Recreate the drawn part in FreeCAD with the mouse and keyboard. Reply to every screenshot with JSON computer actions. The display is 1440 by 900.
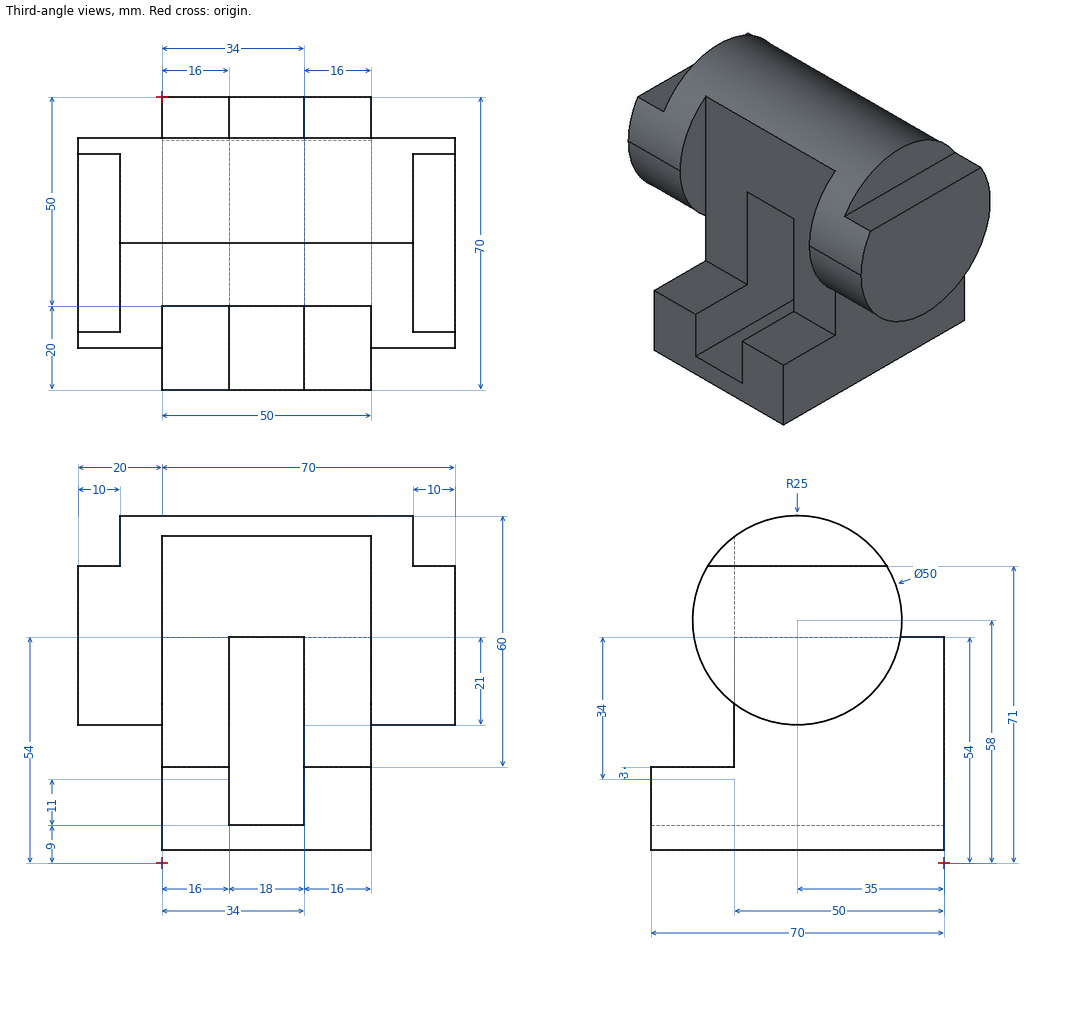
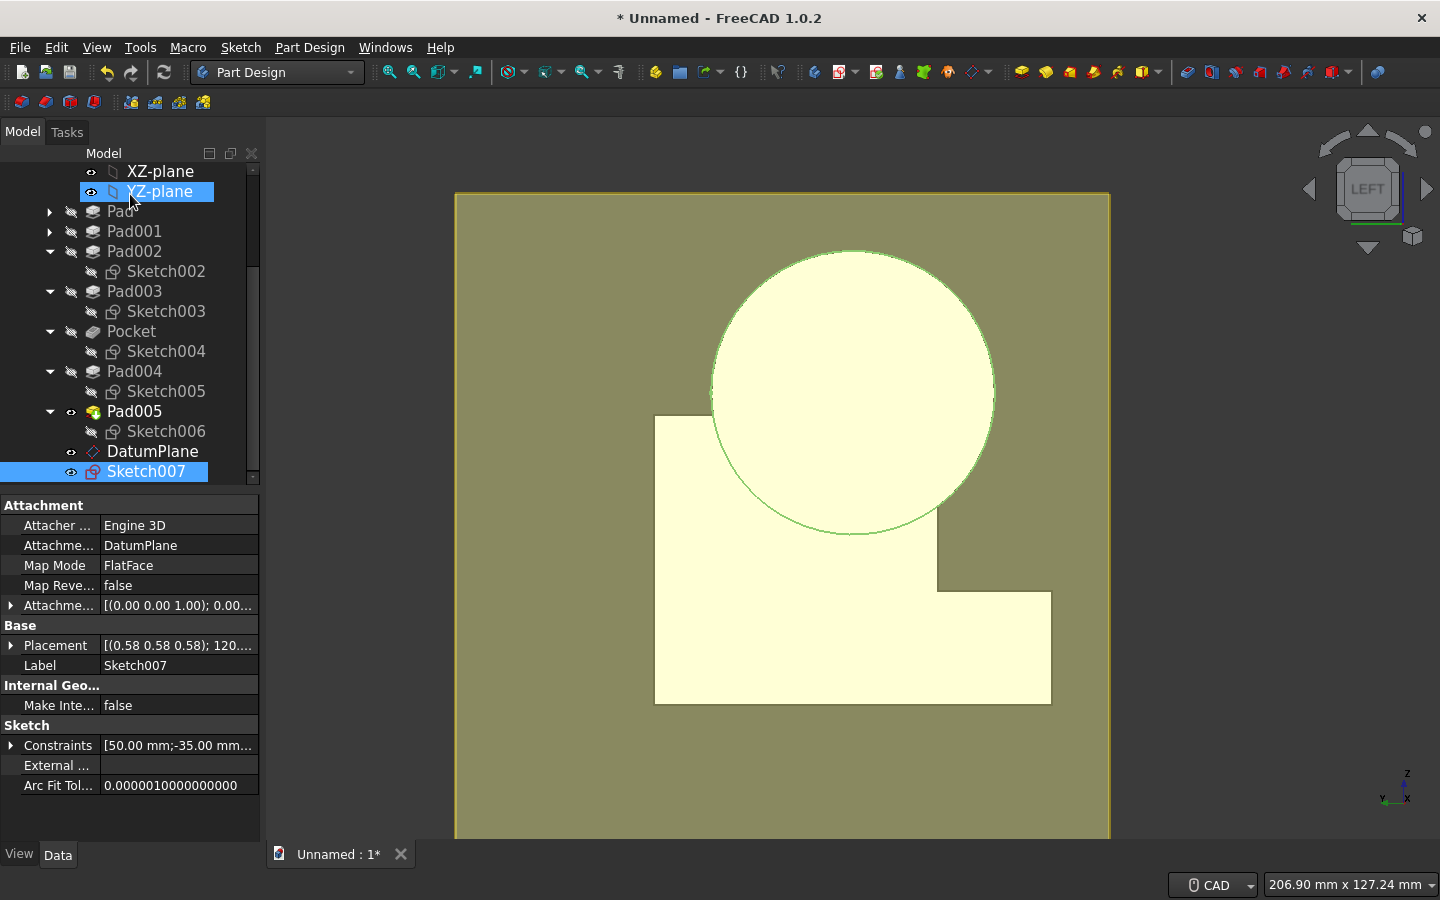
{"action": "left_click", "coordinate": [1022, 72]}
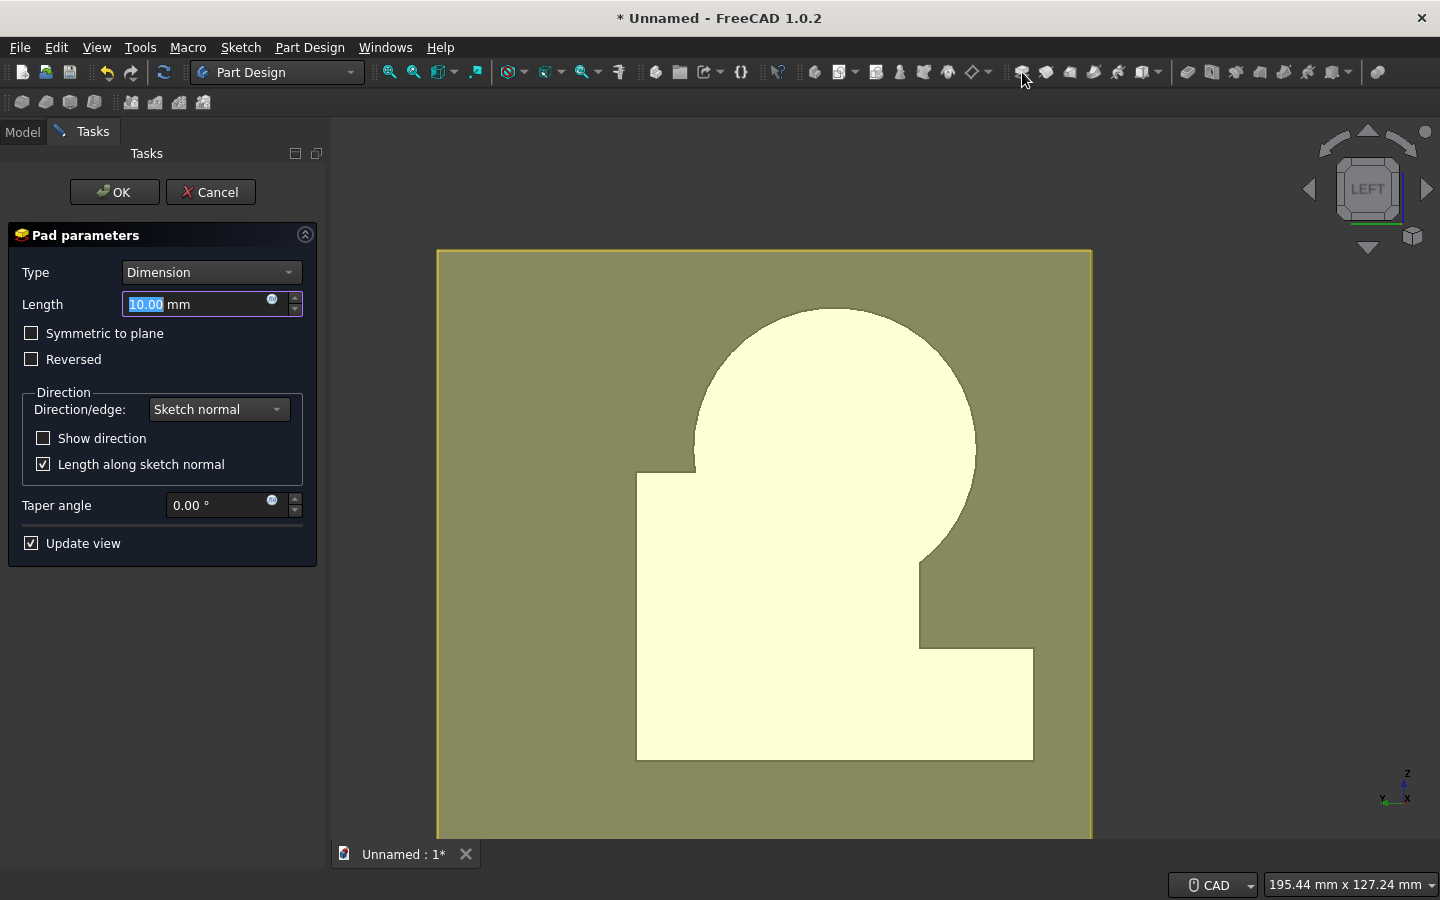
{"action": "type", "text": "20"}
{"action": "key", "text": "Tab"}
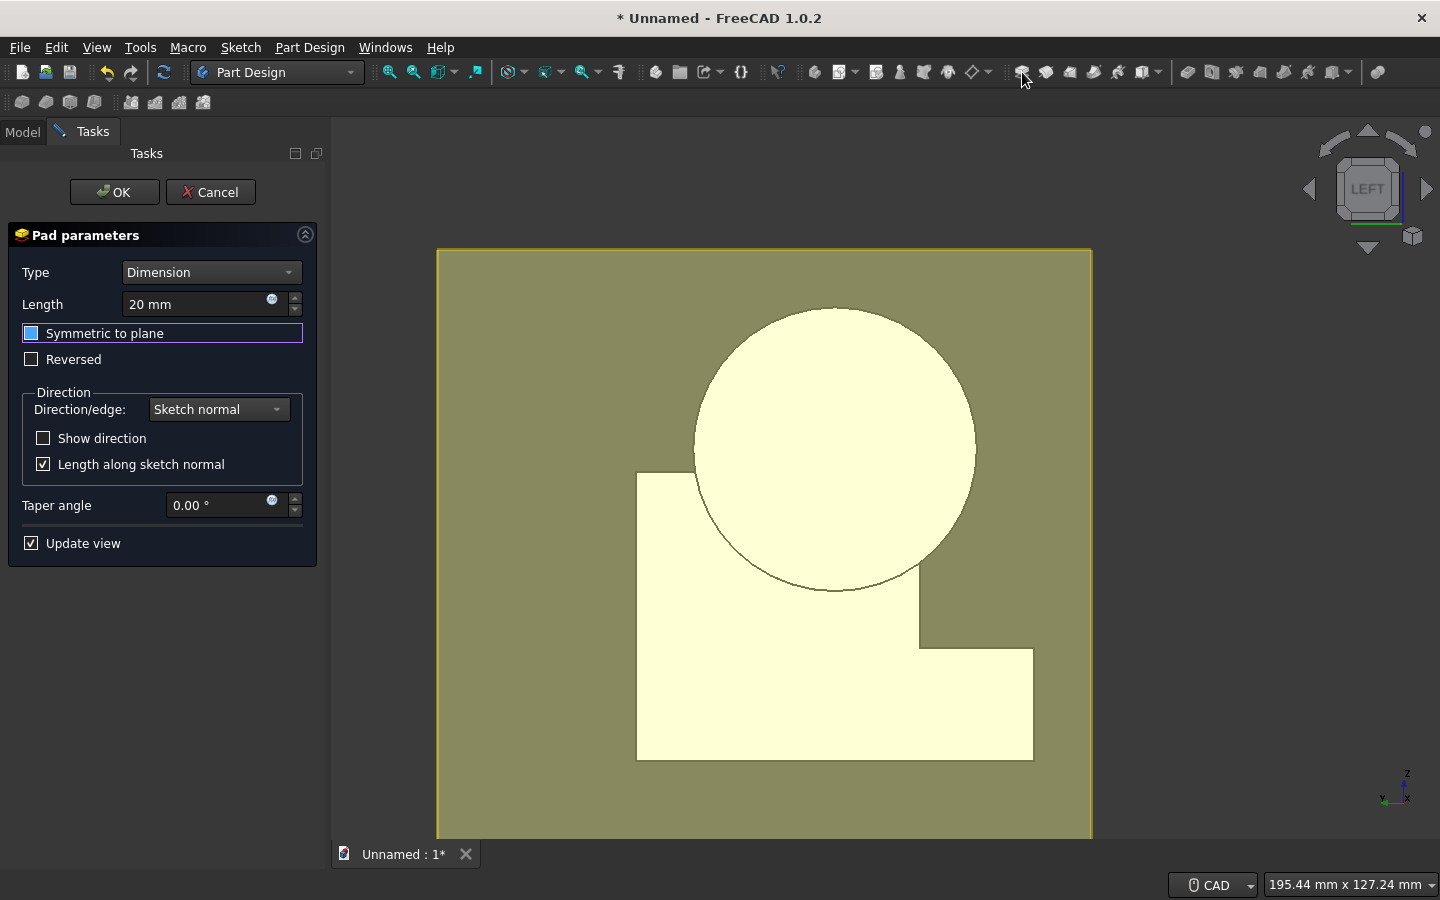
{"action": "left_click", "coordinate": [115, 192]}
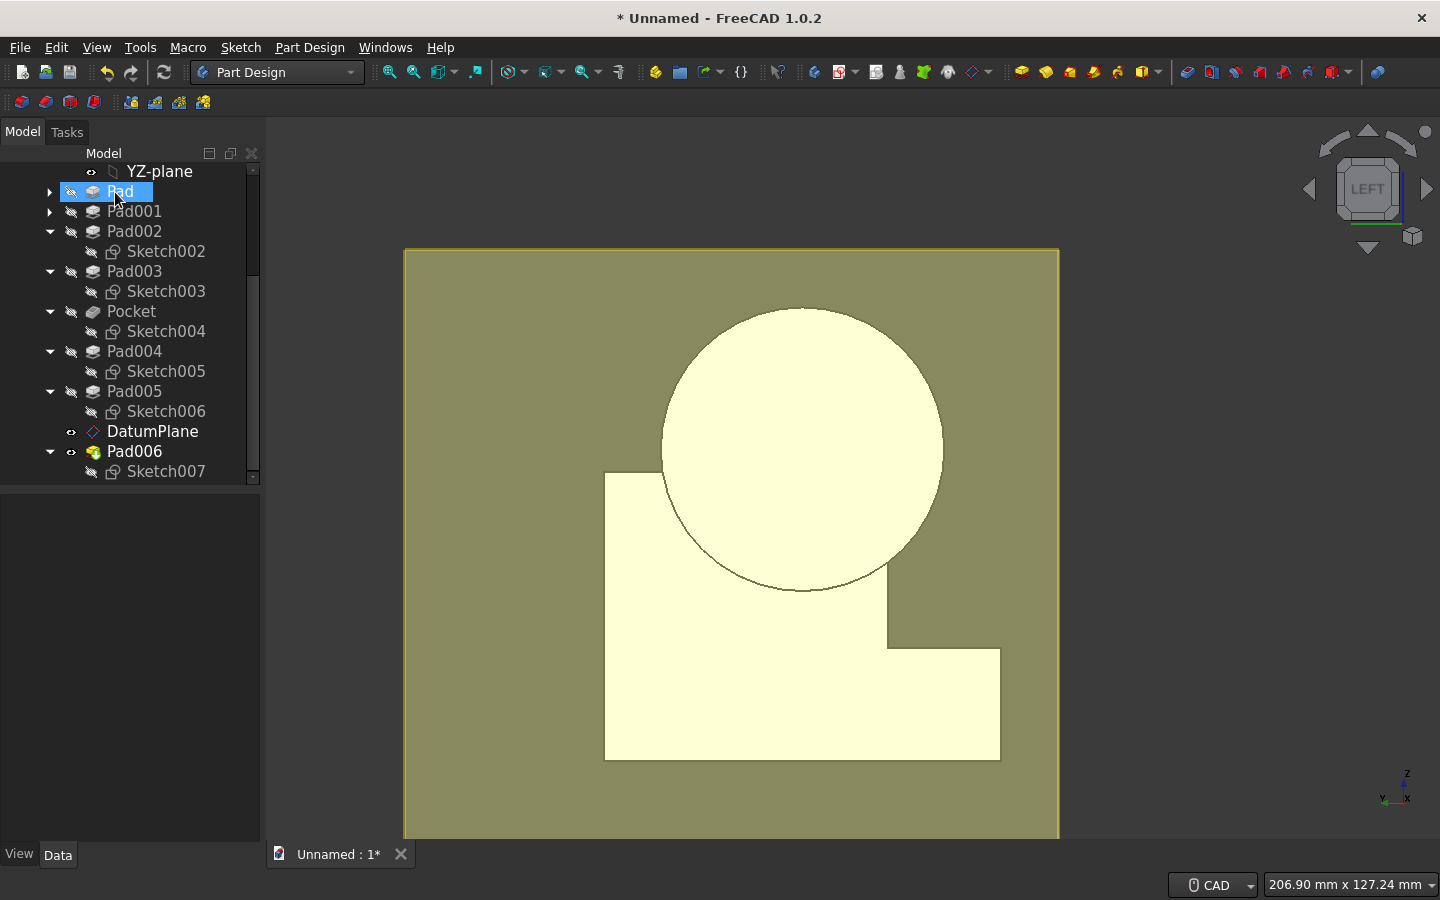
{"action": "left_click", "coordinate": [116, 432]}
{"action": "key", "text": "space"}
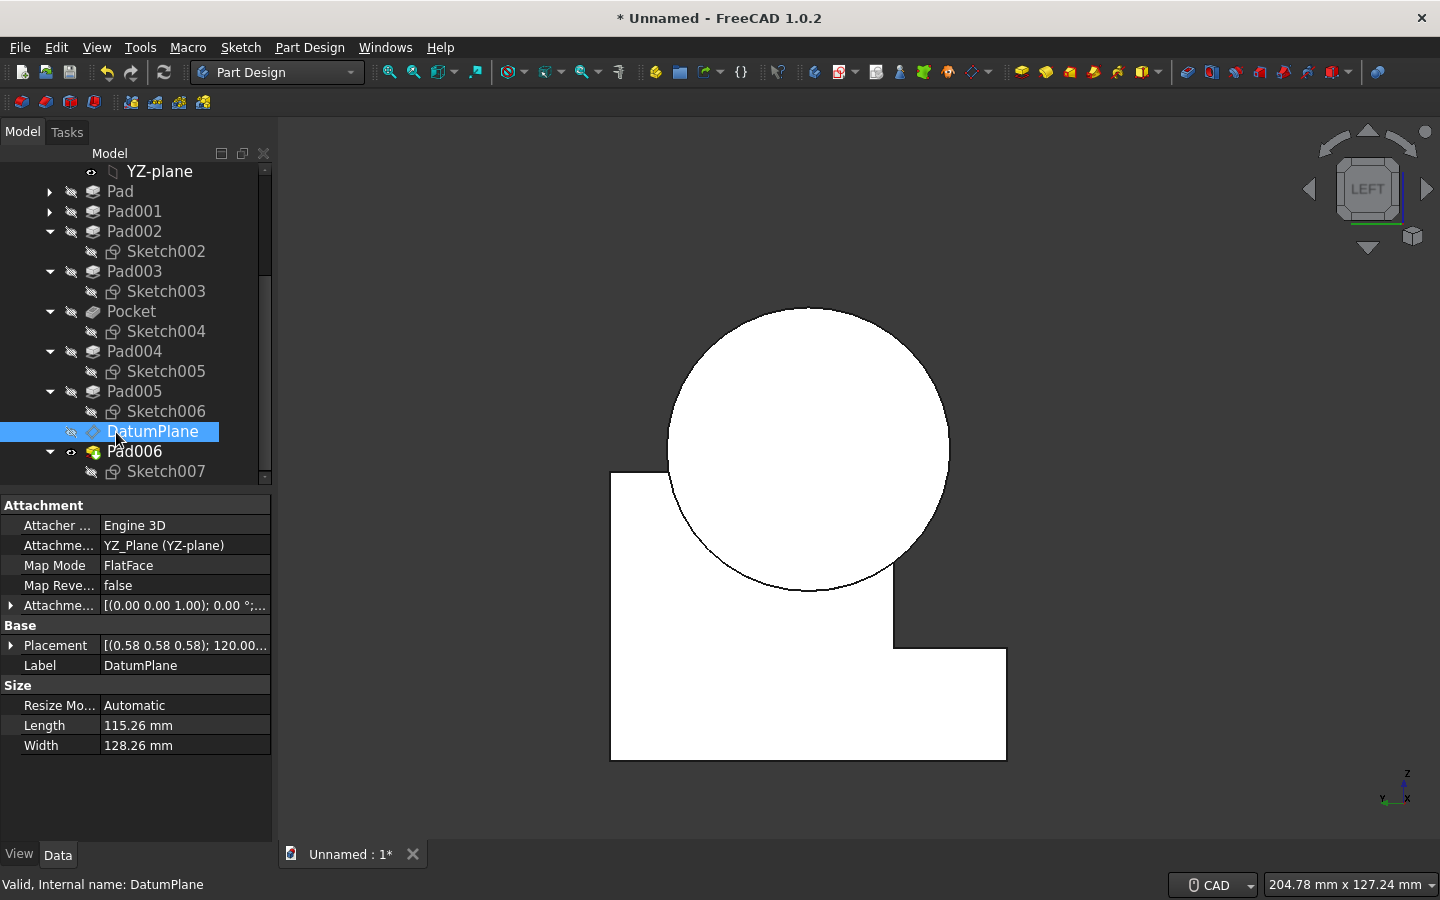
{"action": "key", "text": "0"}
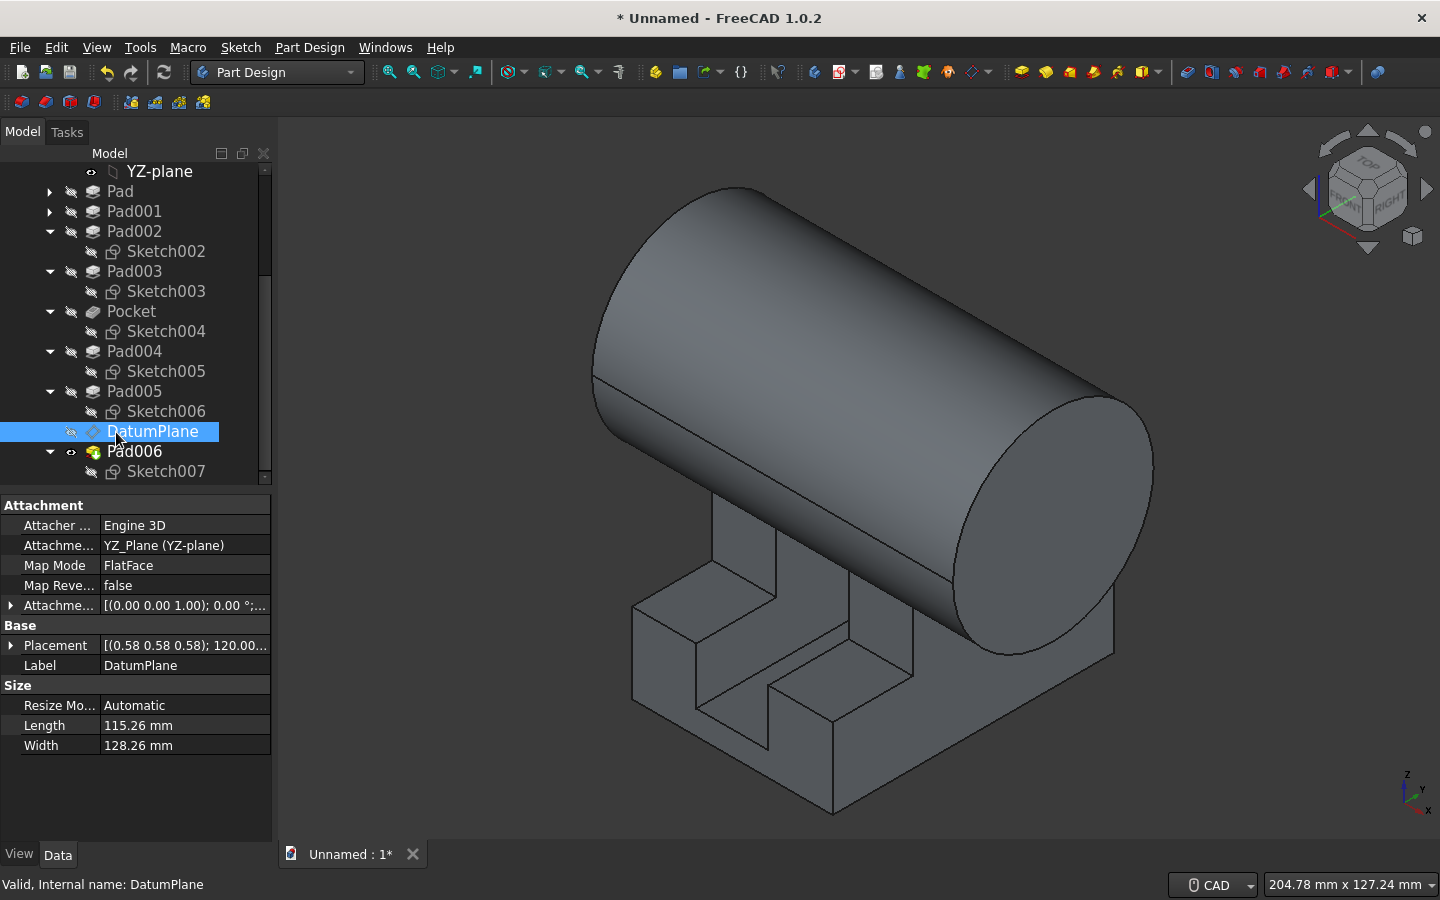
{"action": "key", "text": "v f"}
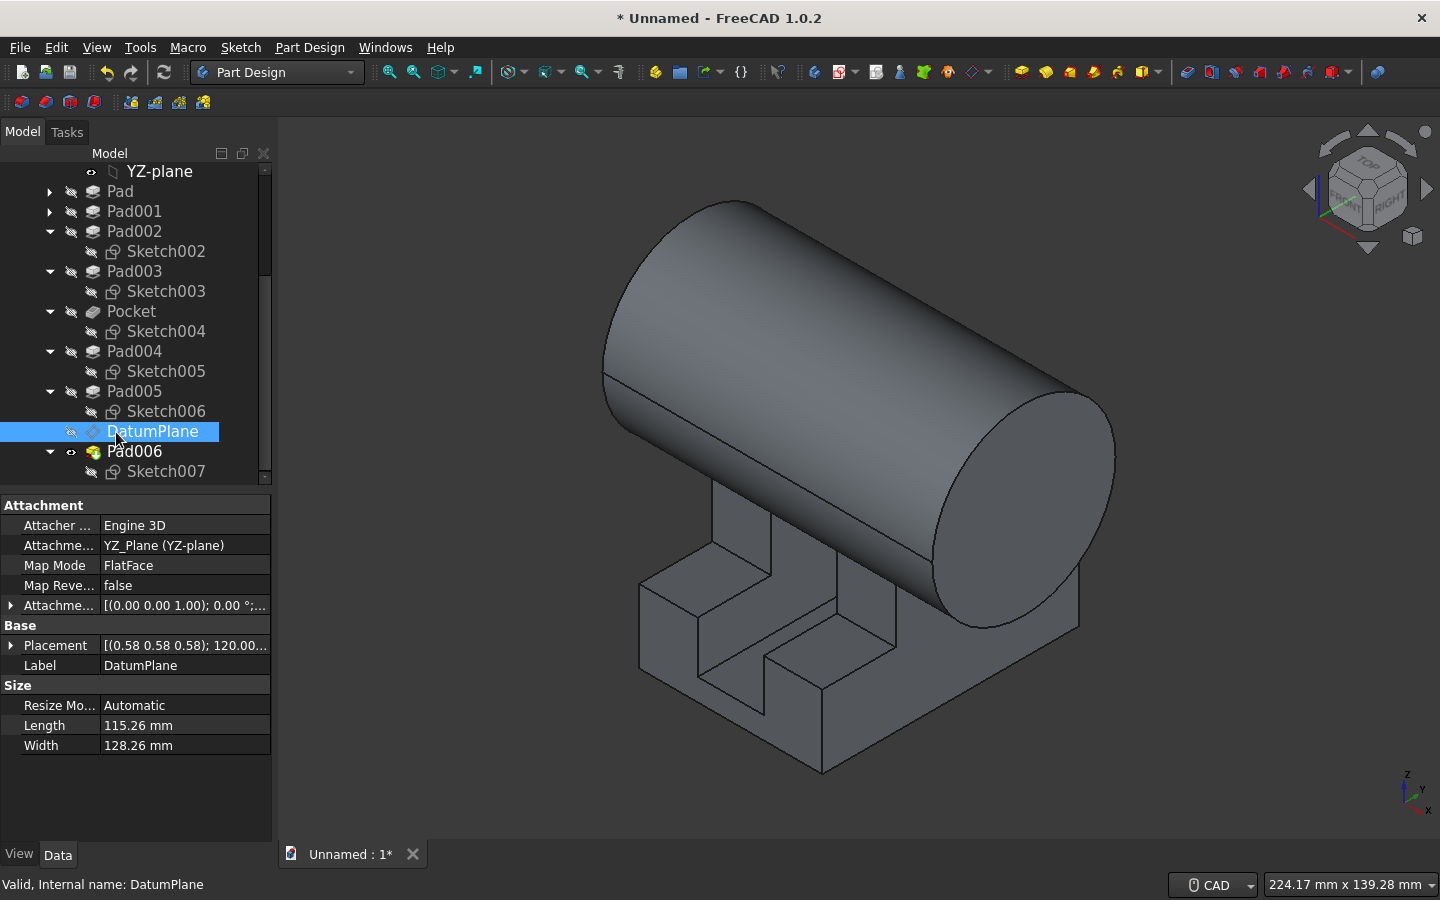
{"action": "left_click", "coordinate": [705, 579]}